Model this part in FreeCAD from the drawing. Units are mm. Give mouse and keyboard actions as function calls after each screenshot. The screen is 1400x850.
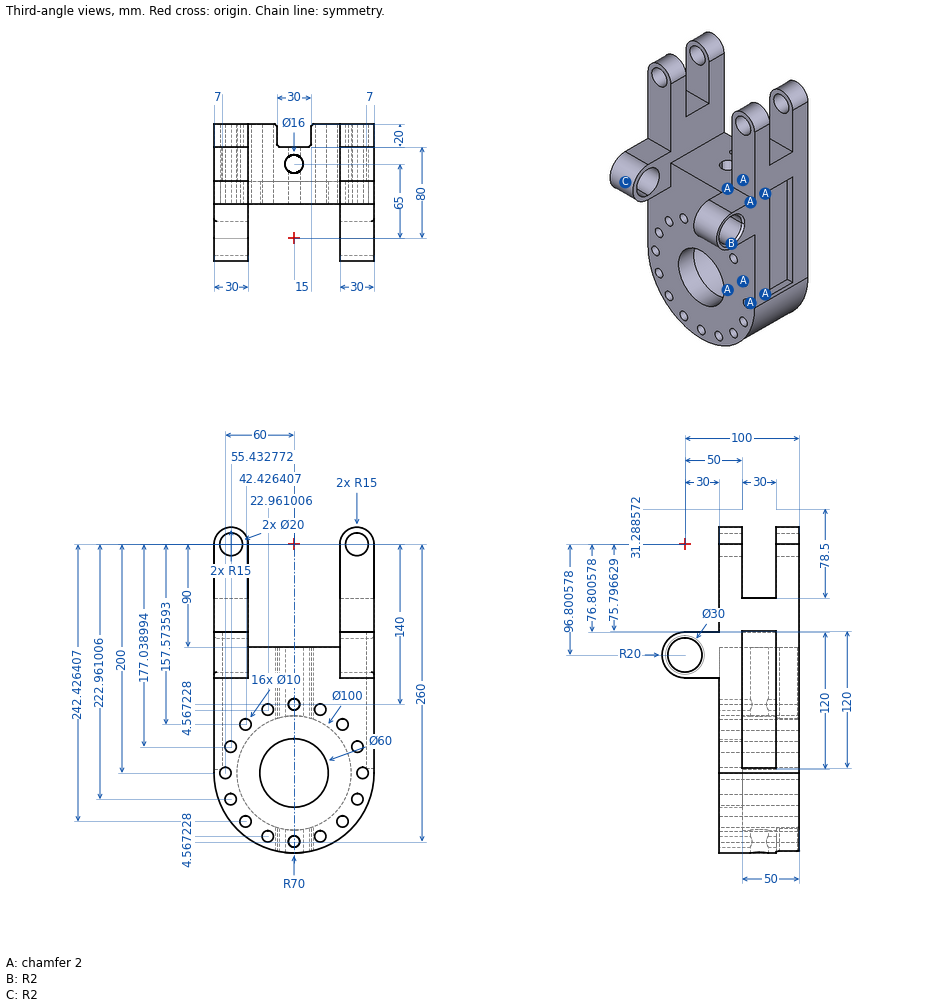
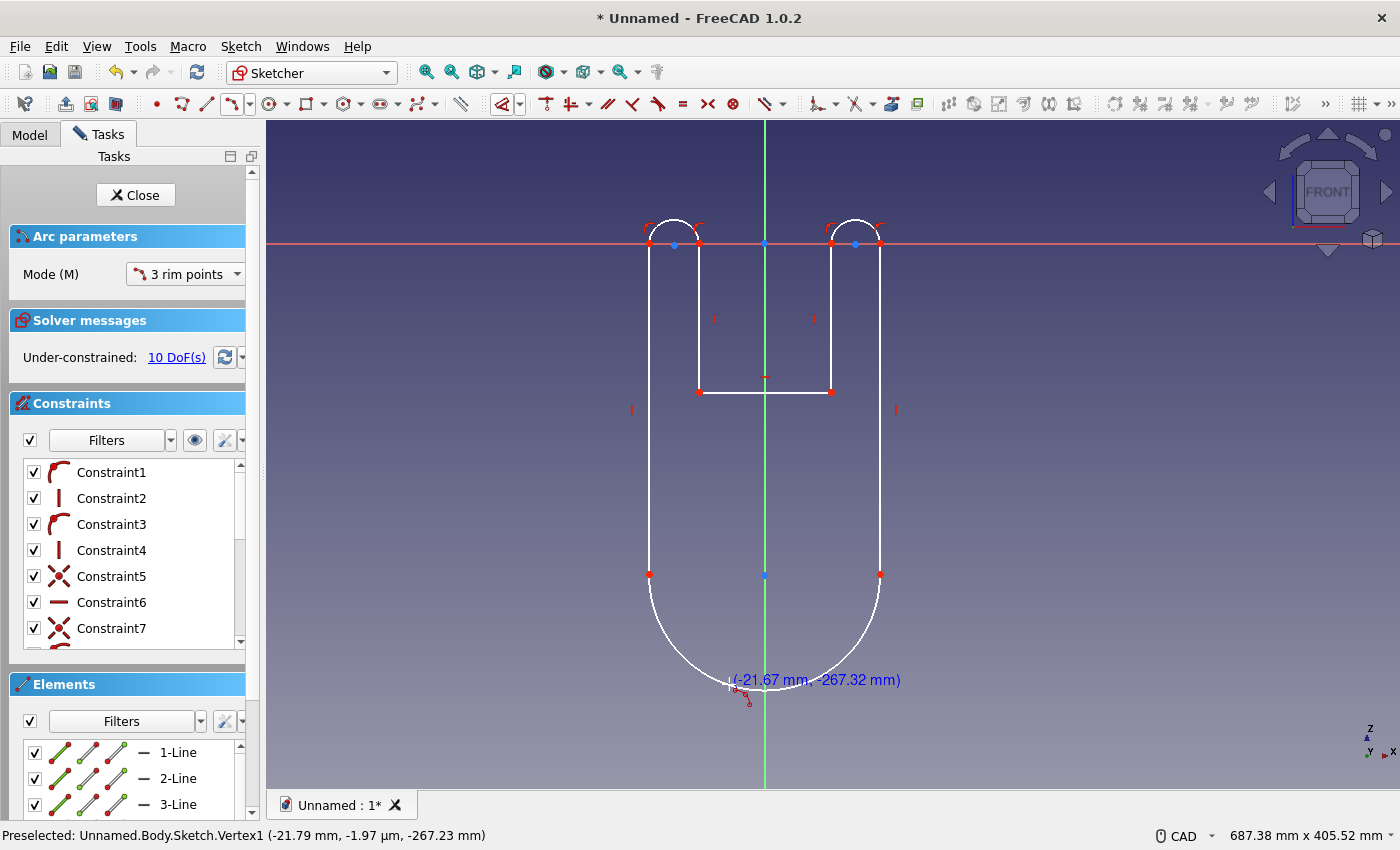
click(268, 104)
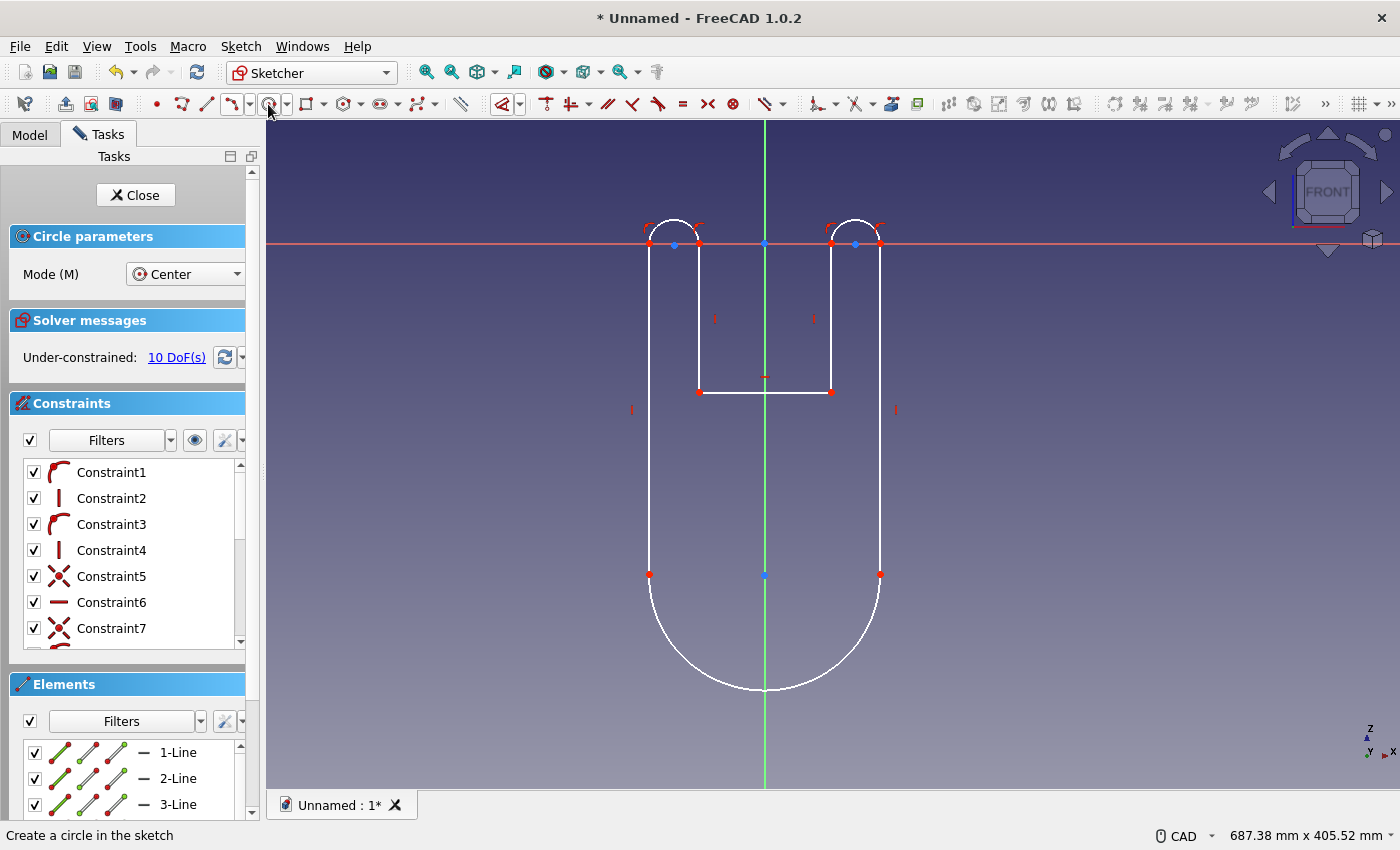
scroll(674, 244, up, 2)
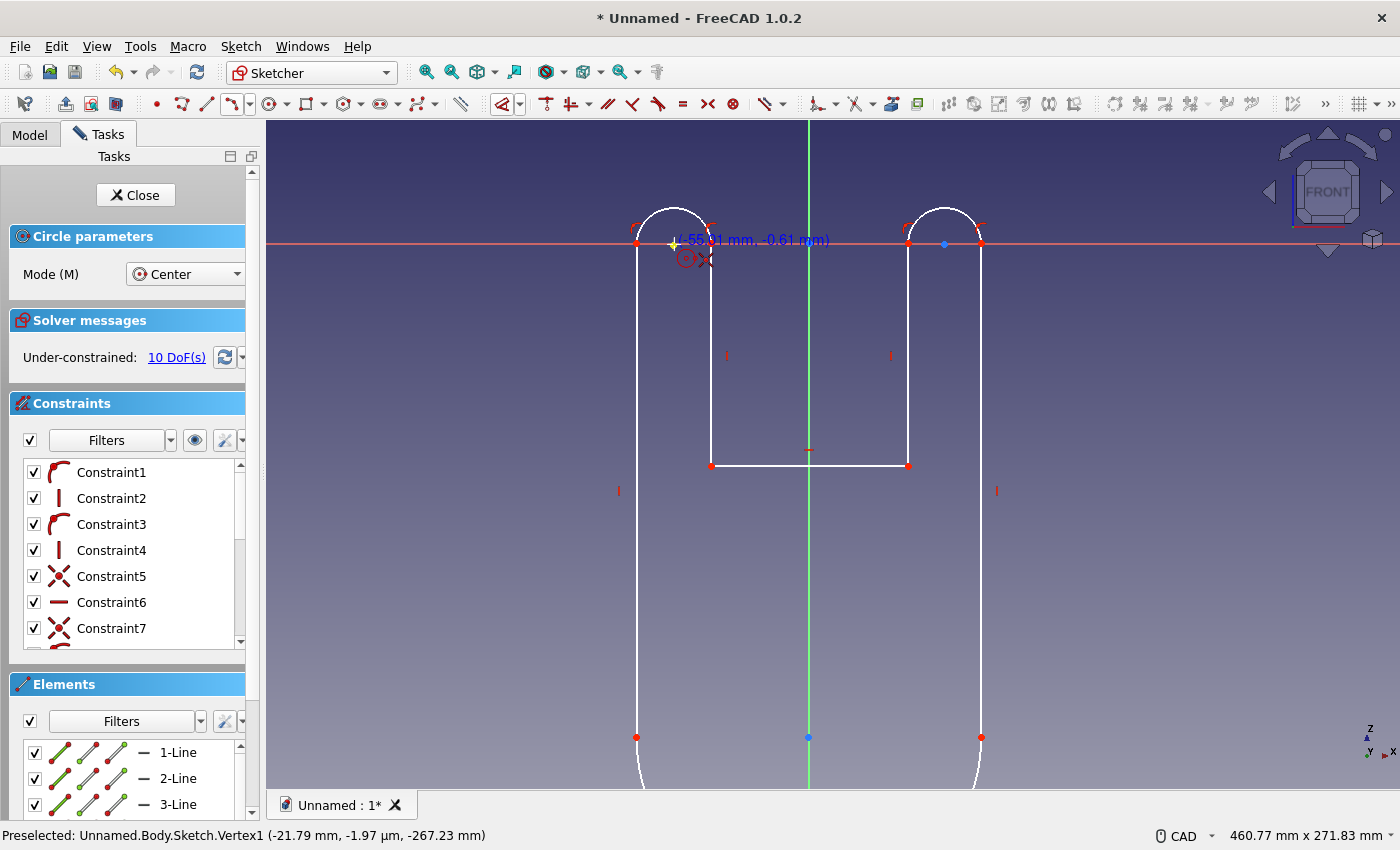
click(674, 244)
click(691, 261)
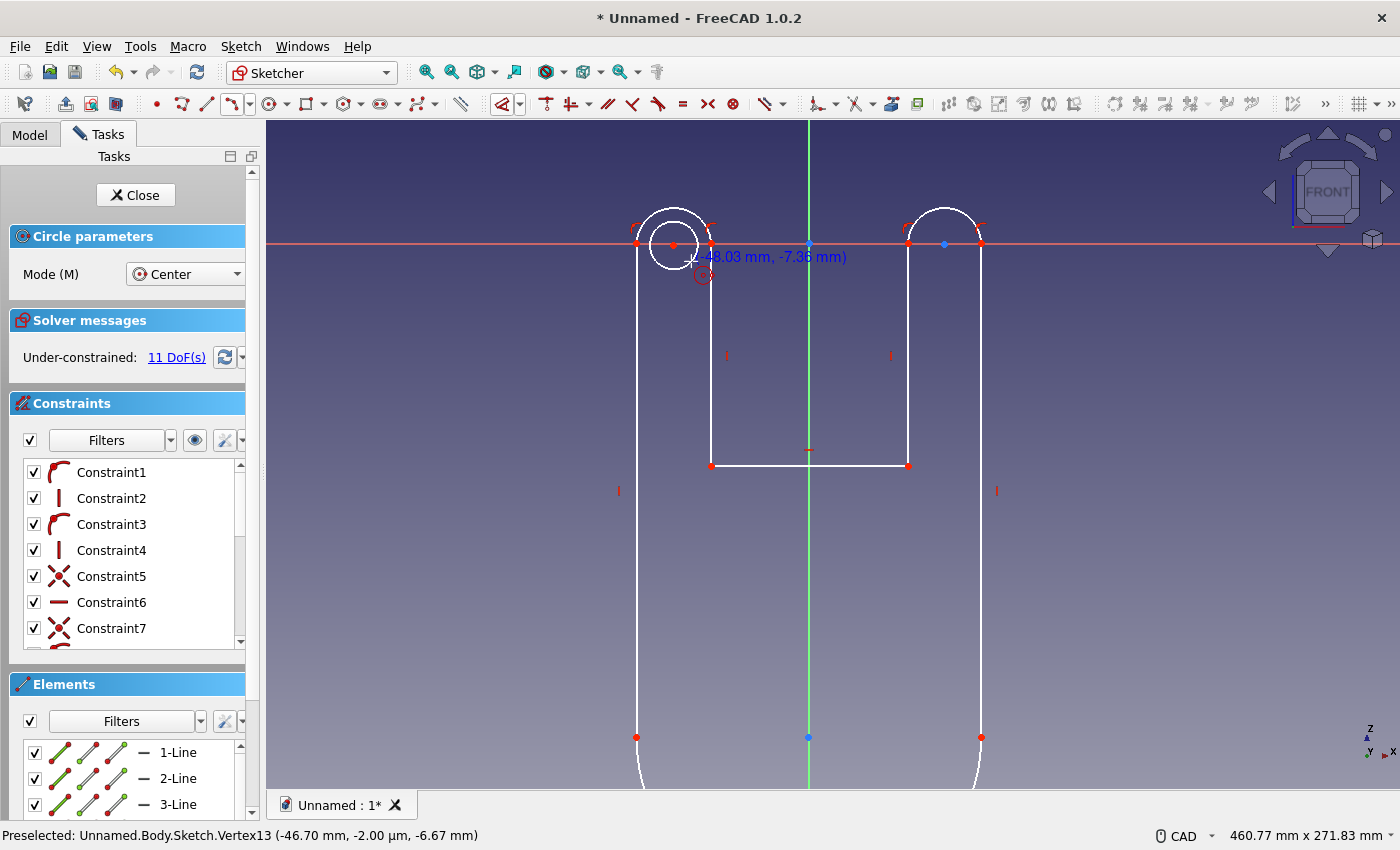
click(945, 244)
click(962, 261)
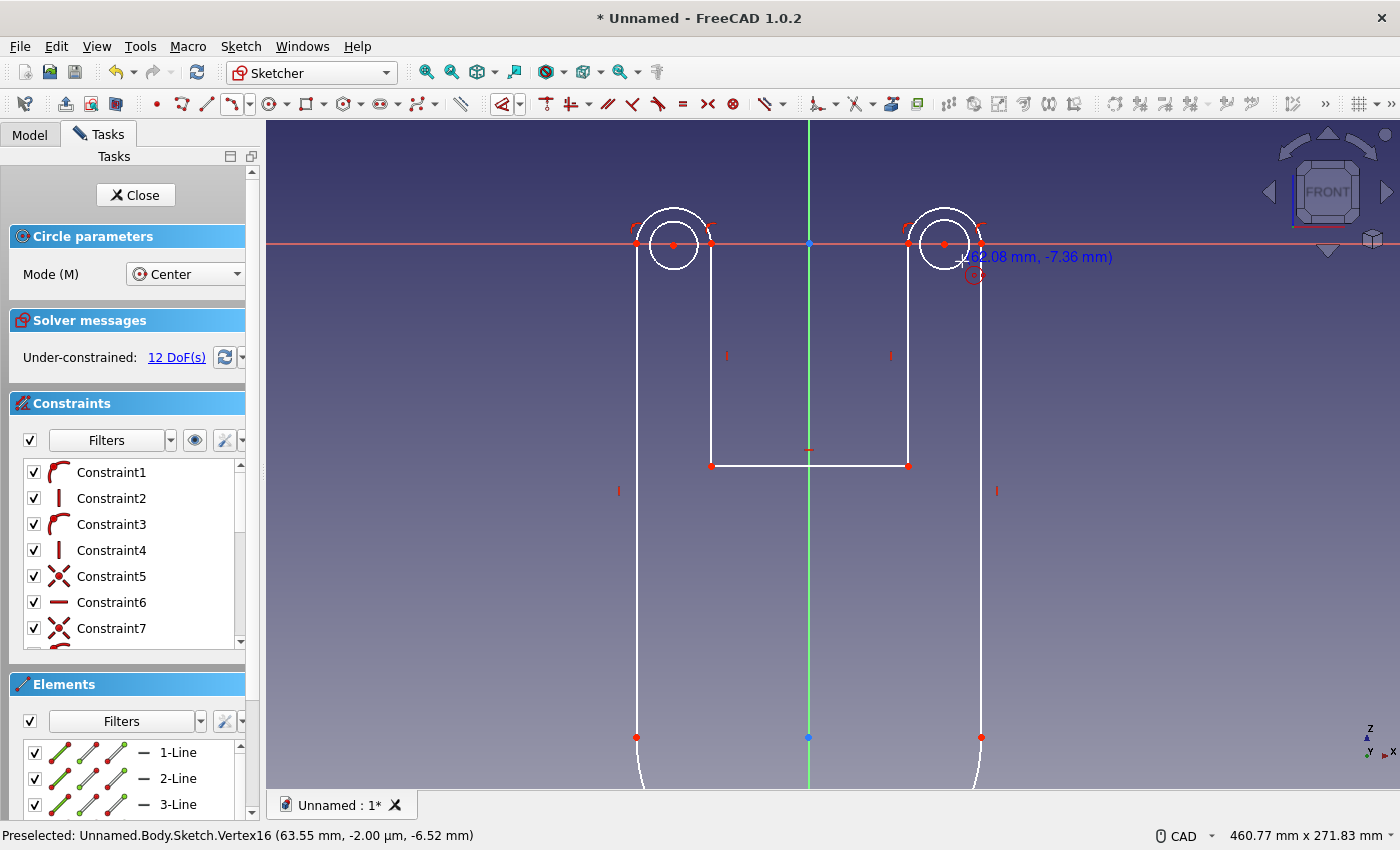
scroll(705, 632, up, 4)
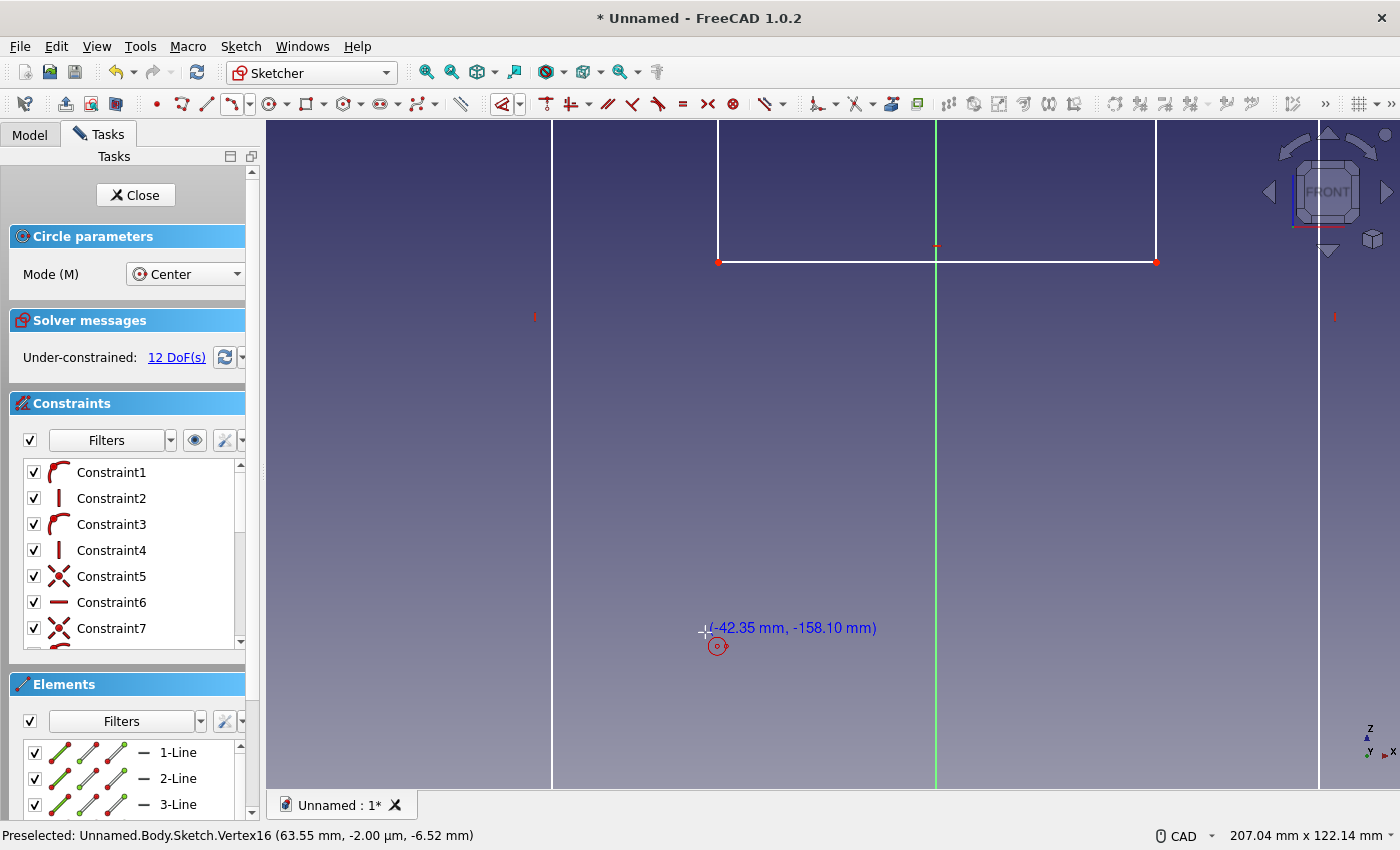
click(704, 630)
click(723, 611)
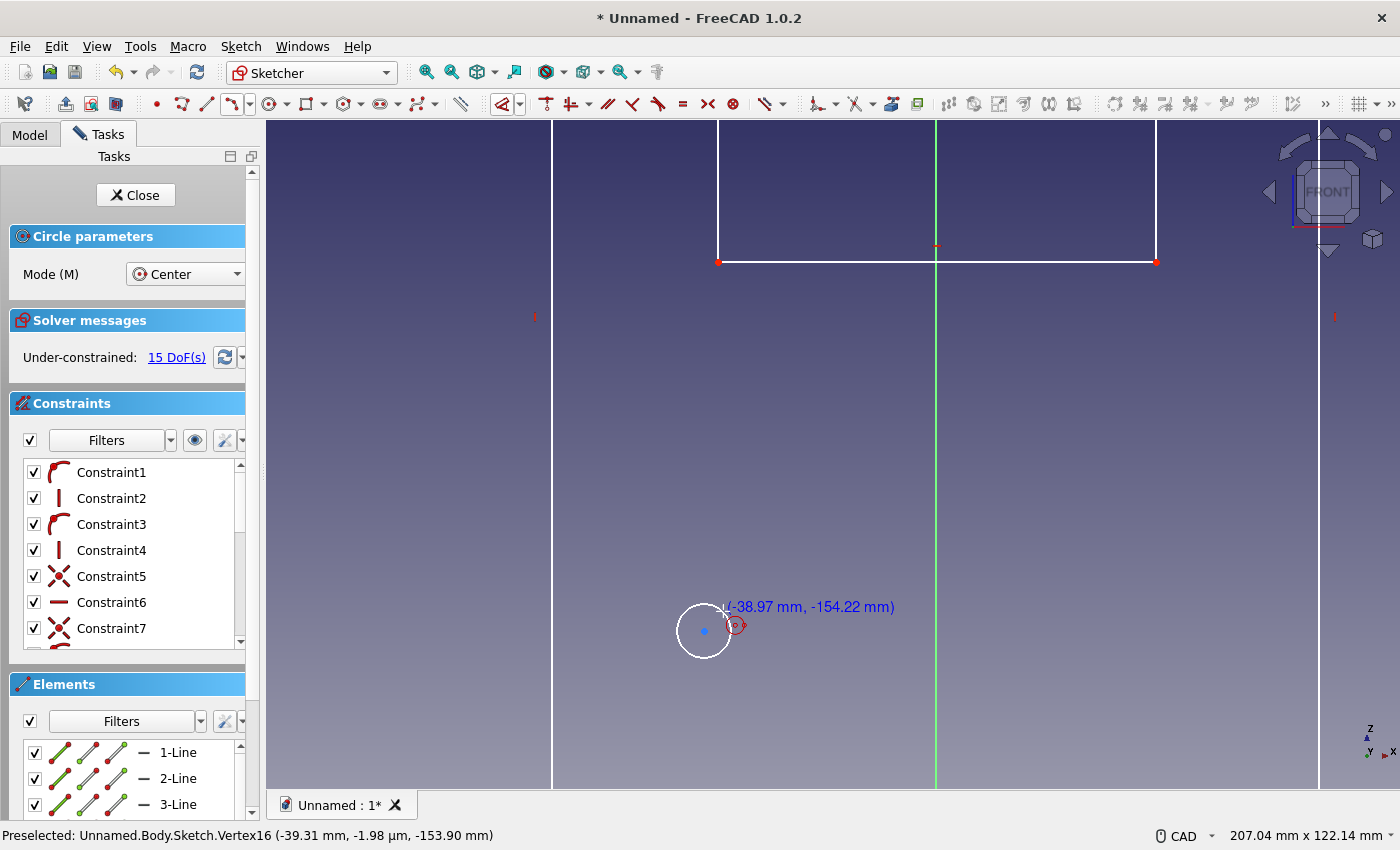
click(633, 737)
click(652, 718)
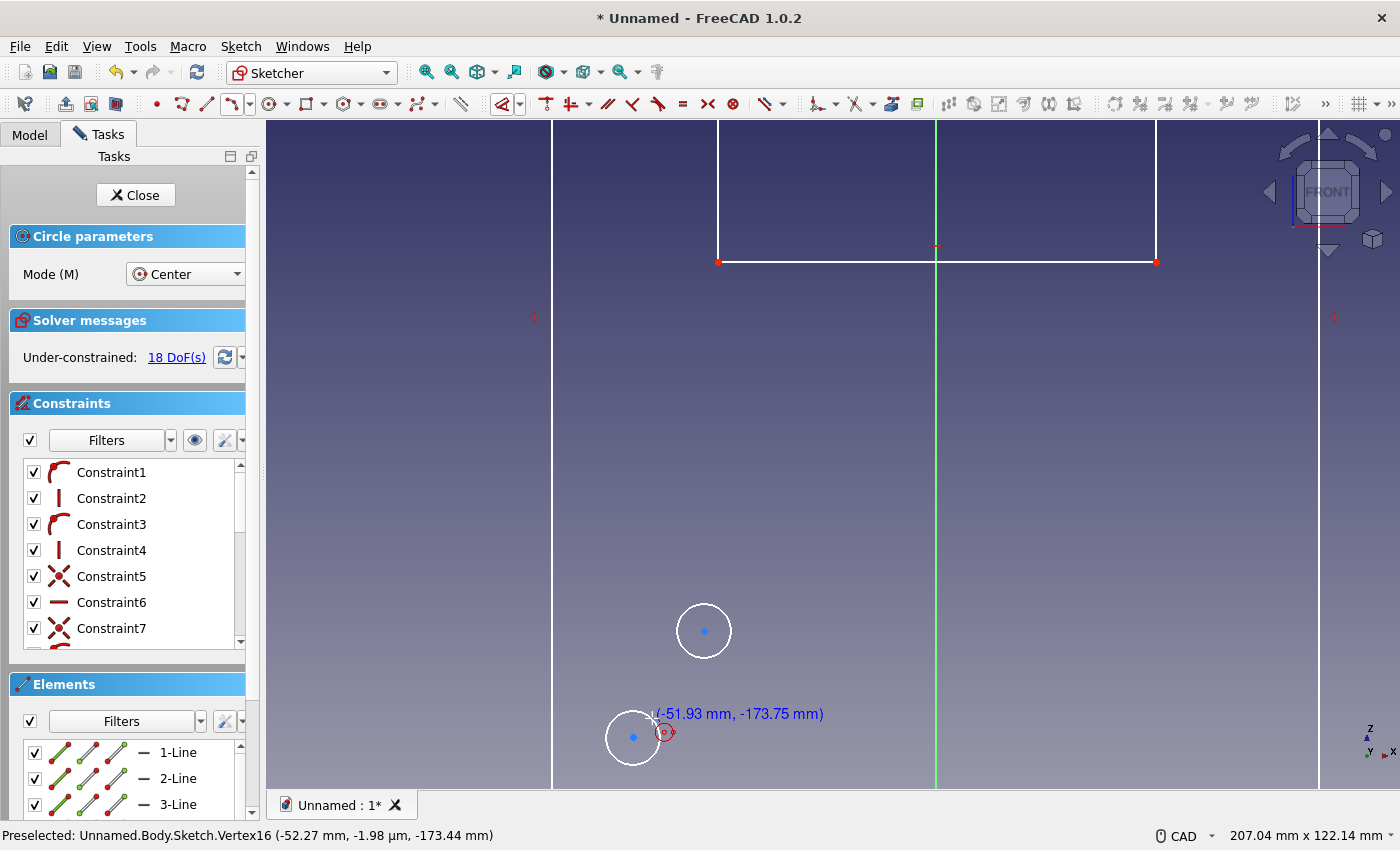
click(811, 559)
click(830, 540)